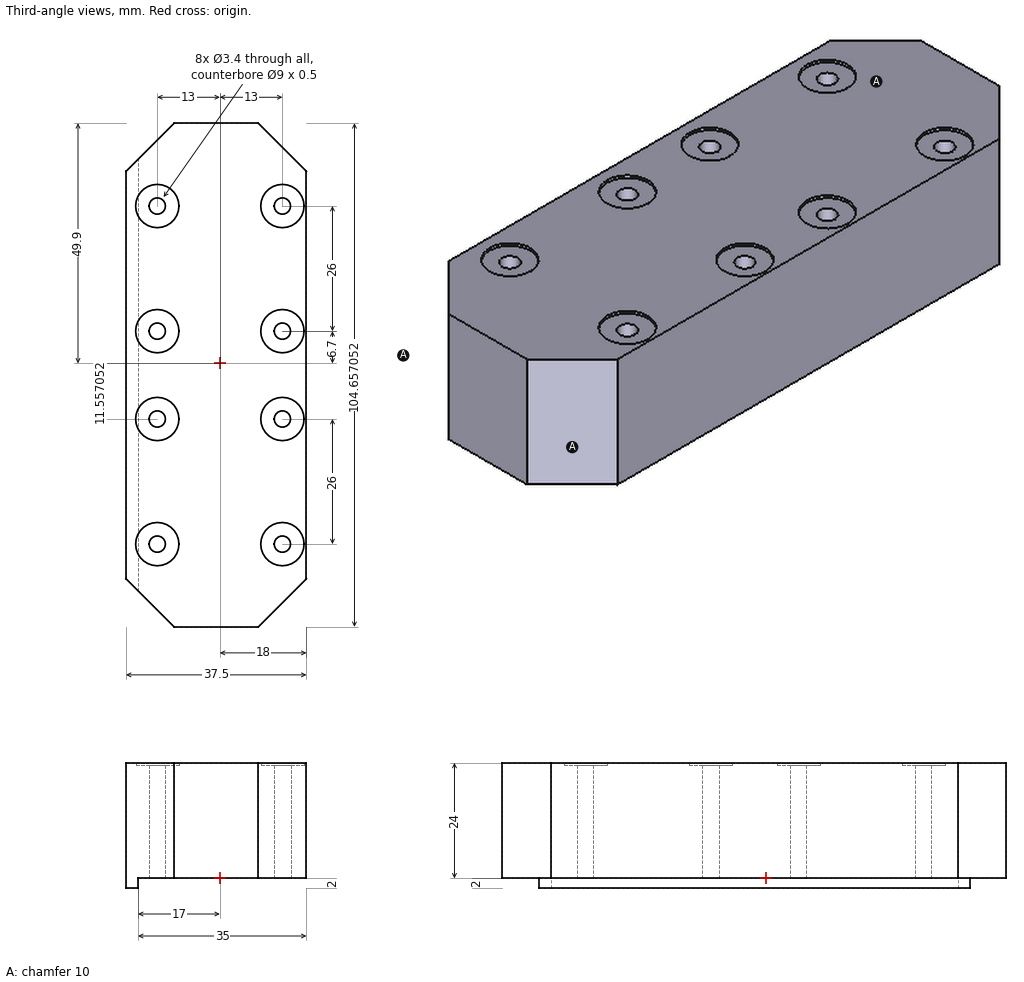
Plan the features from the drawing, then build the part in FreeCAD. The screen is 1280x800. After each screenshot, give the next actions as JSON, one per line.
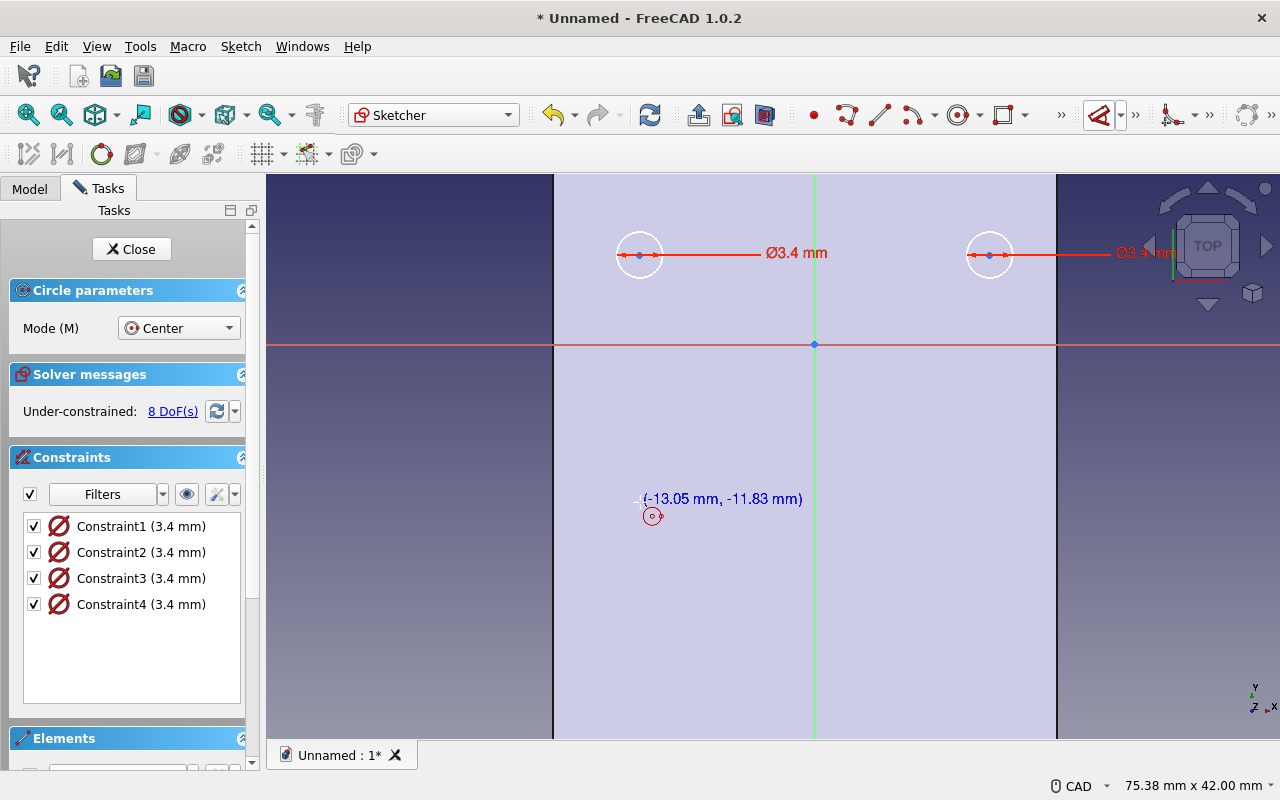
{"action": "left_click", "coordinate": [640, 500]}
{"action": "mouse_move", "coordinate": [656, 484]}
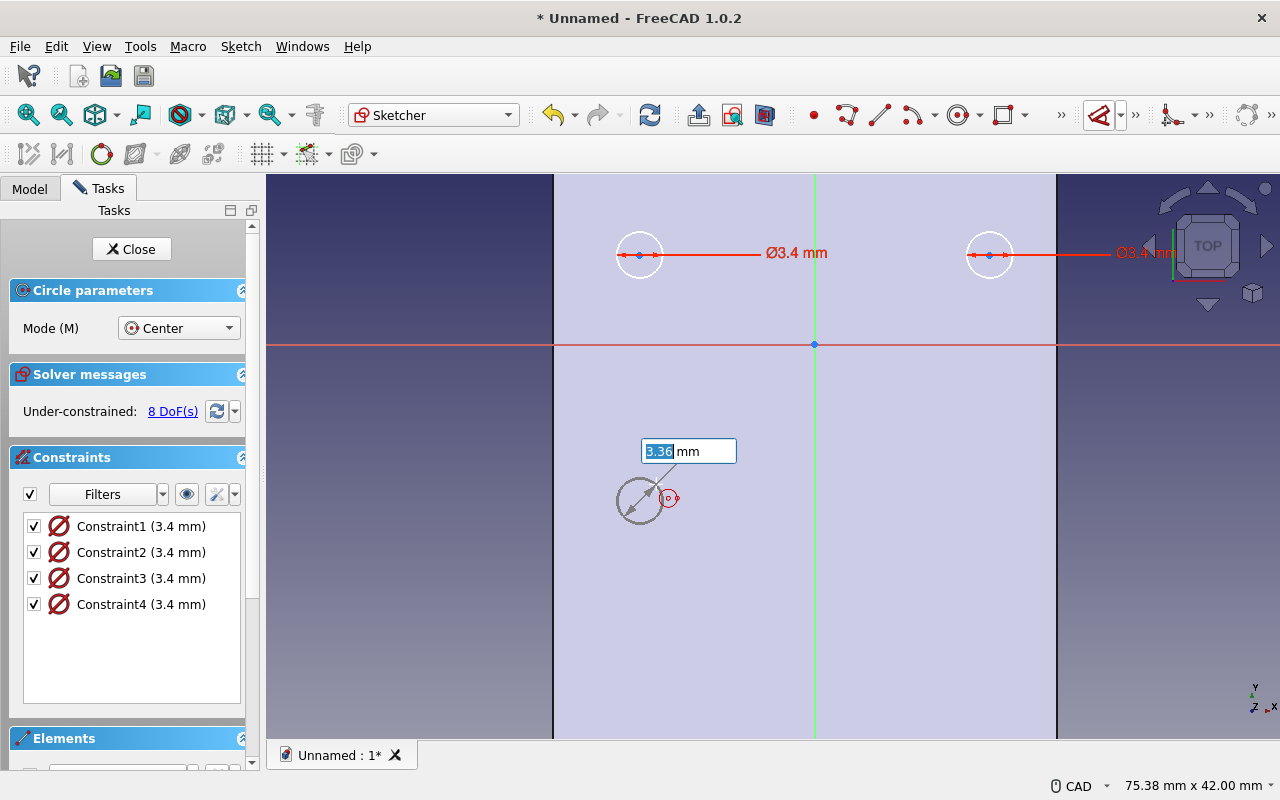
{"action": "type", "text": "3.4"}
{"action": "key", "text": "Return"}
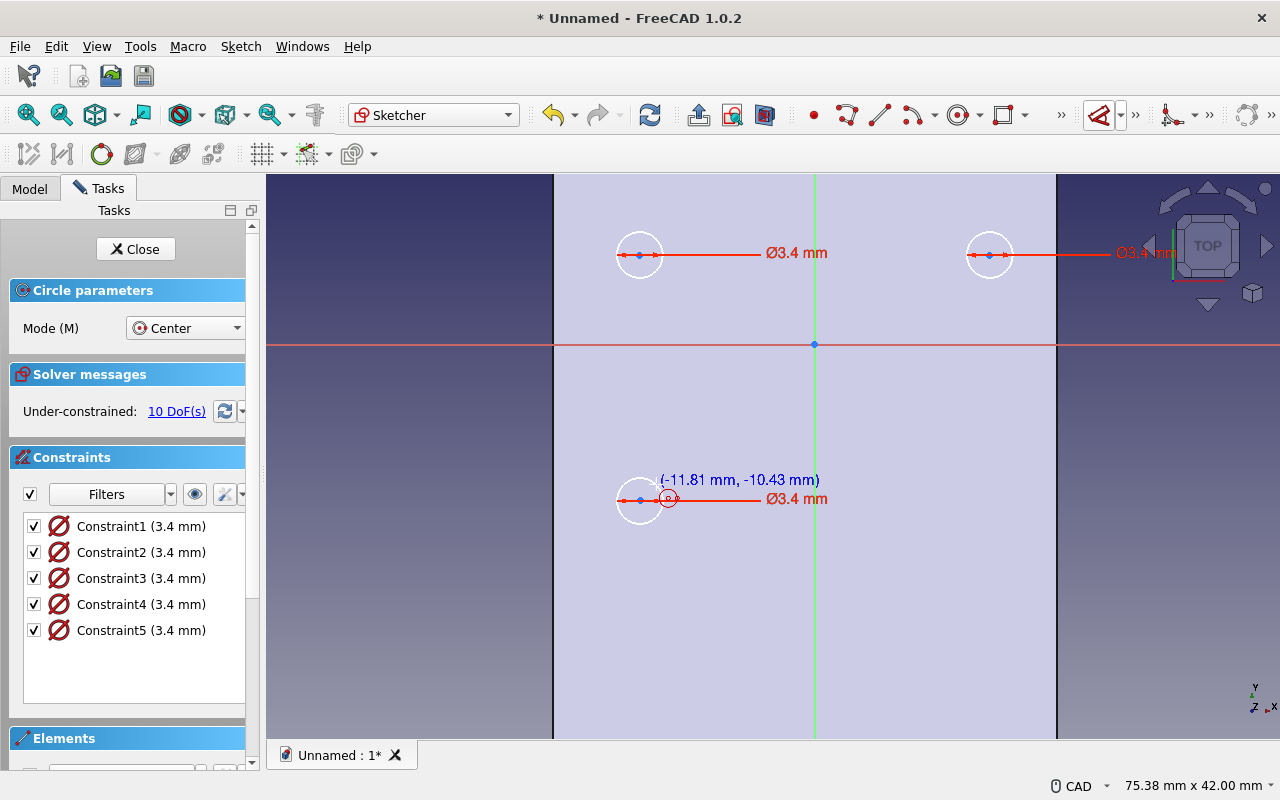
{"action": "left_click", "coordinate": [990, 500]}
{"action": "mouse_move", "coordinate": [1006, 484]}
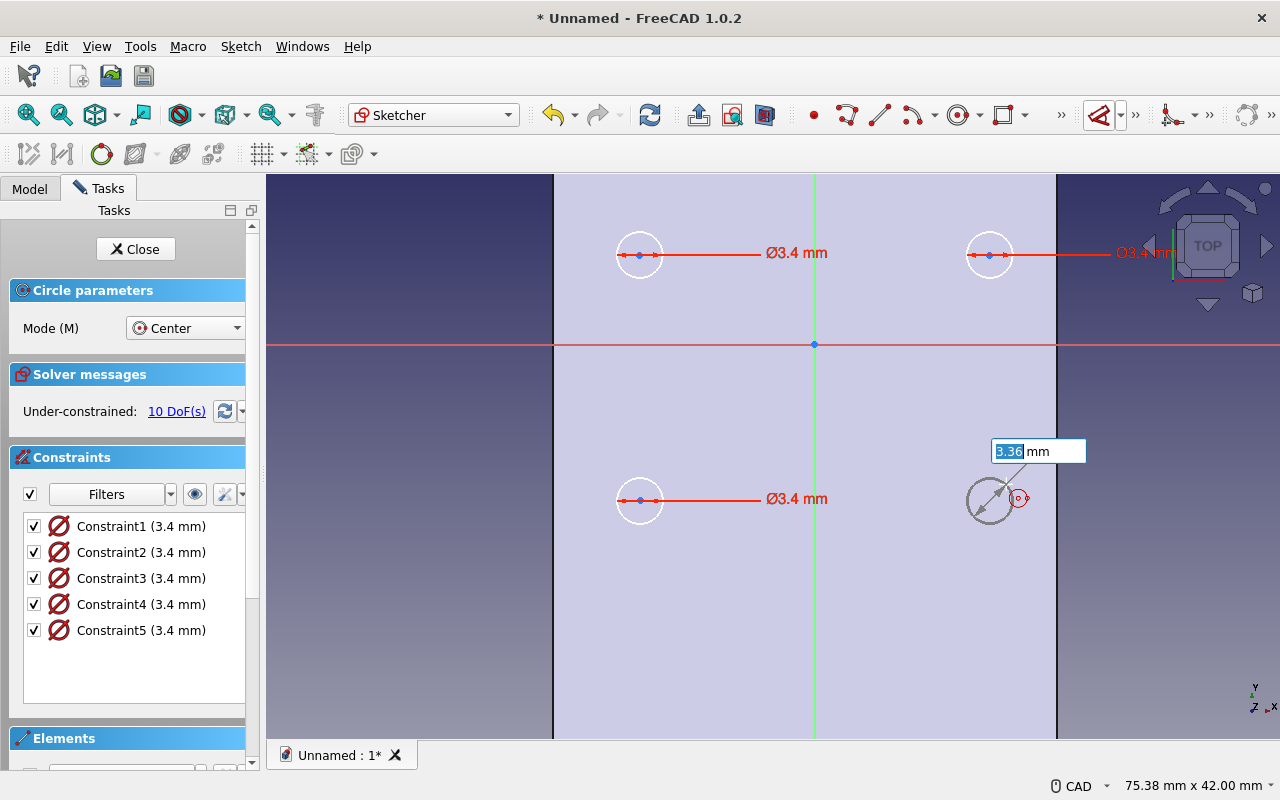
{"action": "type", "text": "3.4"}
{"action": "key", "text": "Return"}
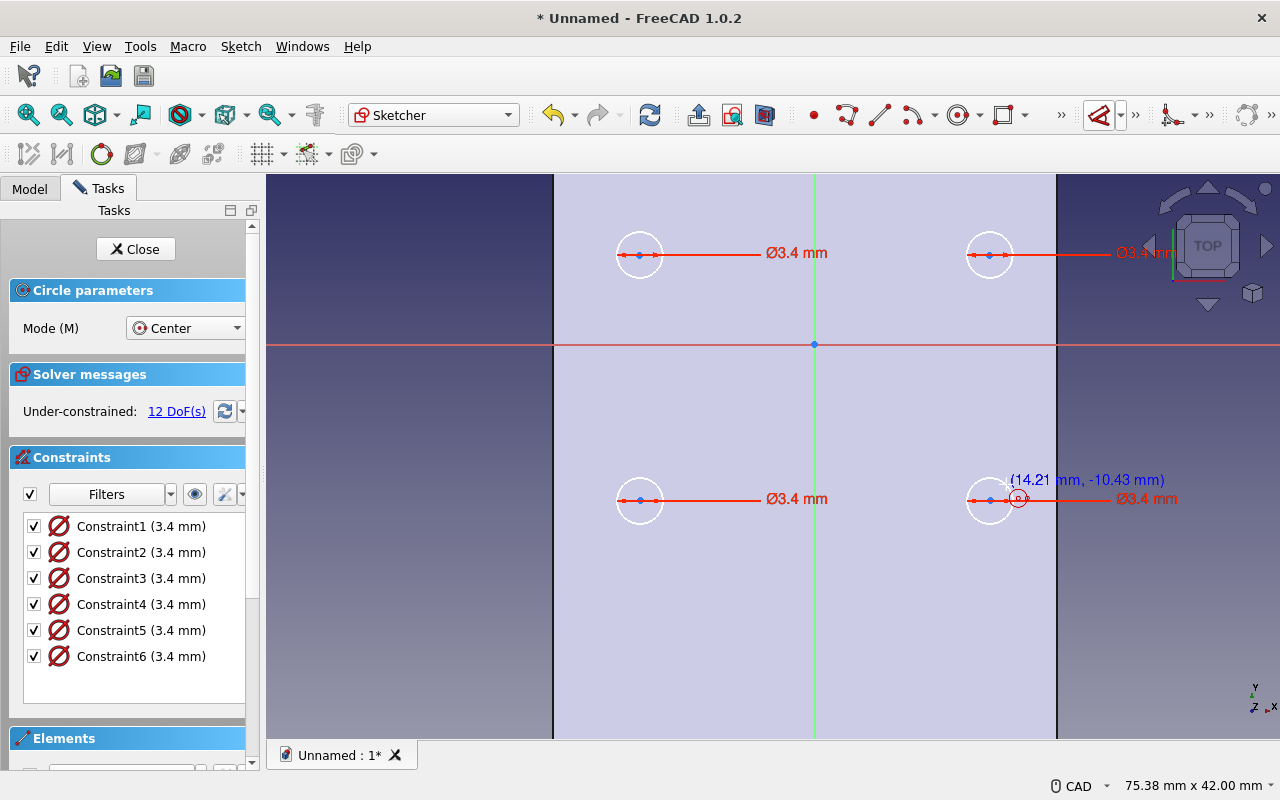
{"action": "scroll", "coordinate": [640, 503], "scroll_direction": "down", "scroll_amount": 5}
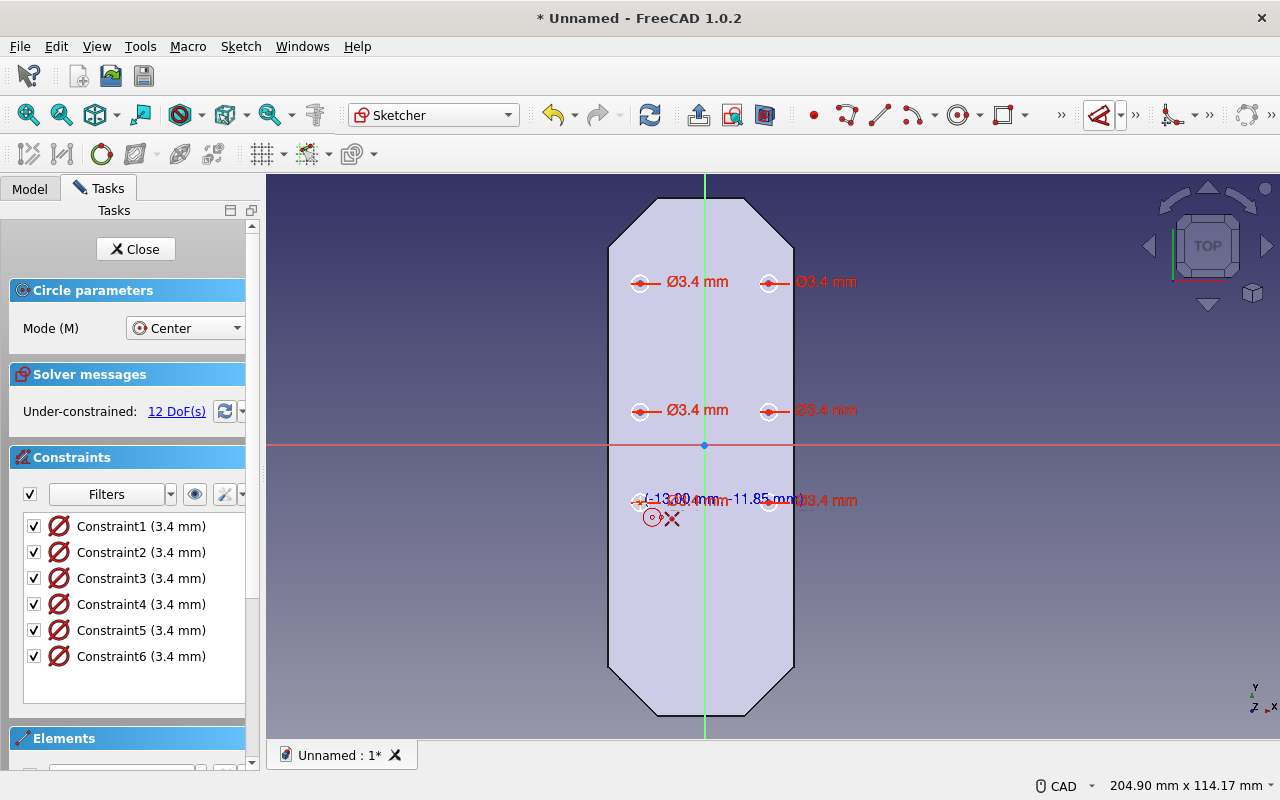
{"action": "scroll", "coordinate": [769, 631], "scroll_direction": "up", "scroll_amount": 5}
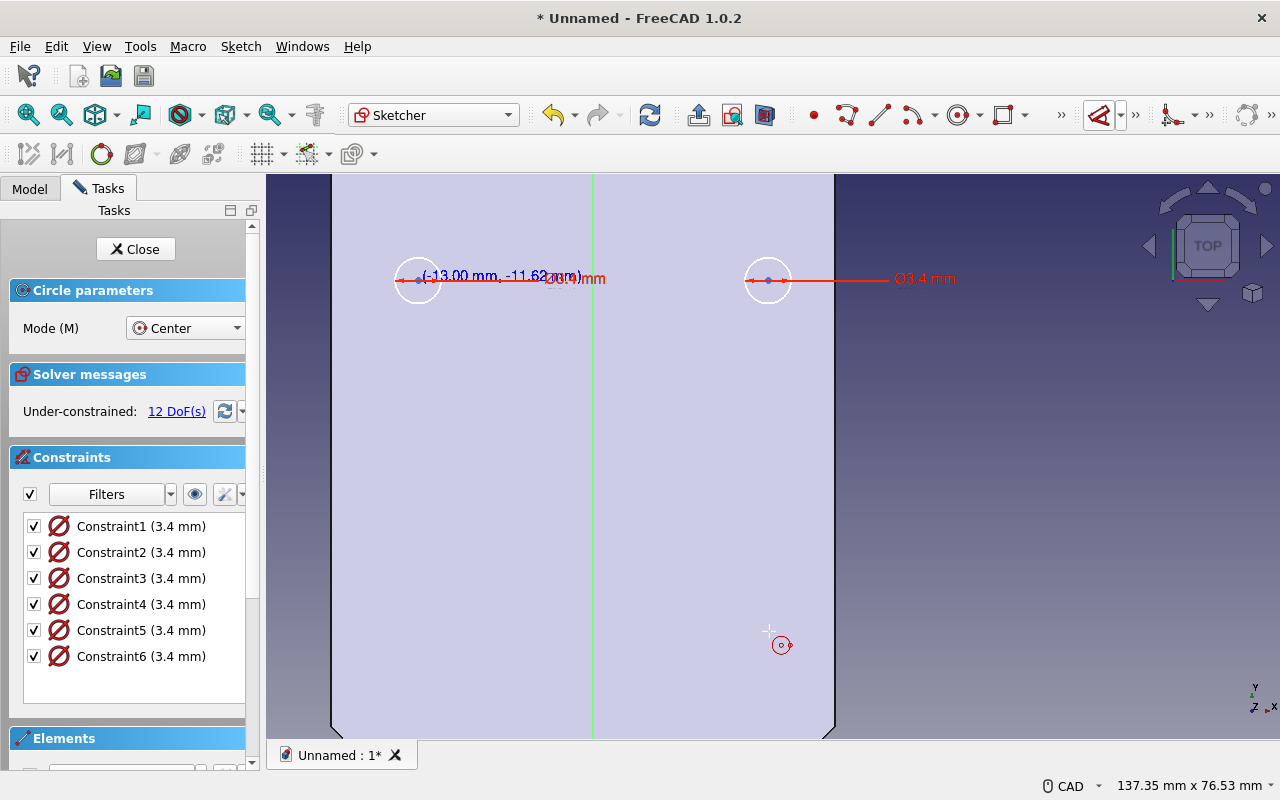
{"action": "left_click", "coordinate": [768, 630]}
{"action": "mouse_move", "coordinate": [784, 613]}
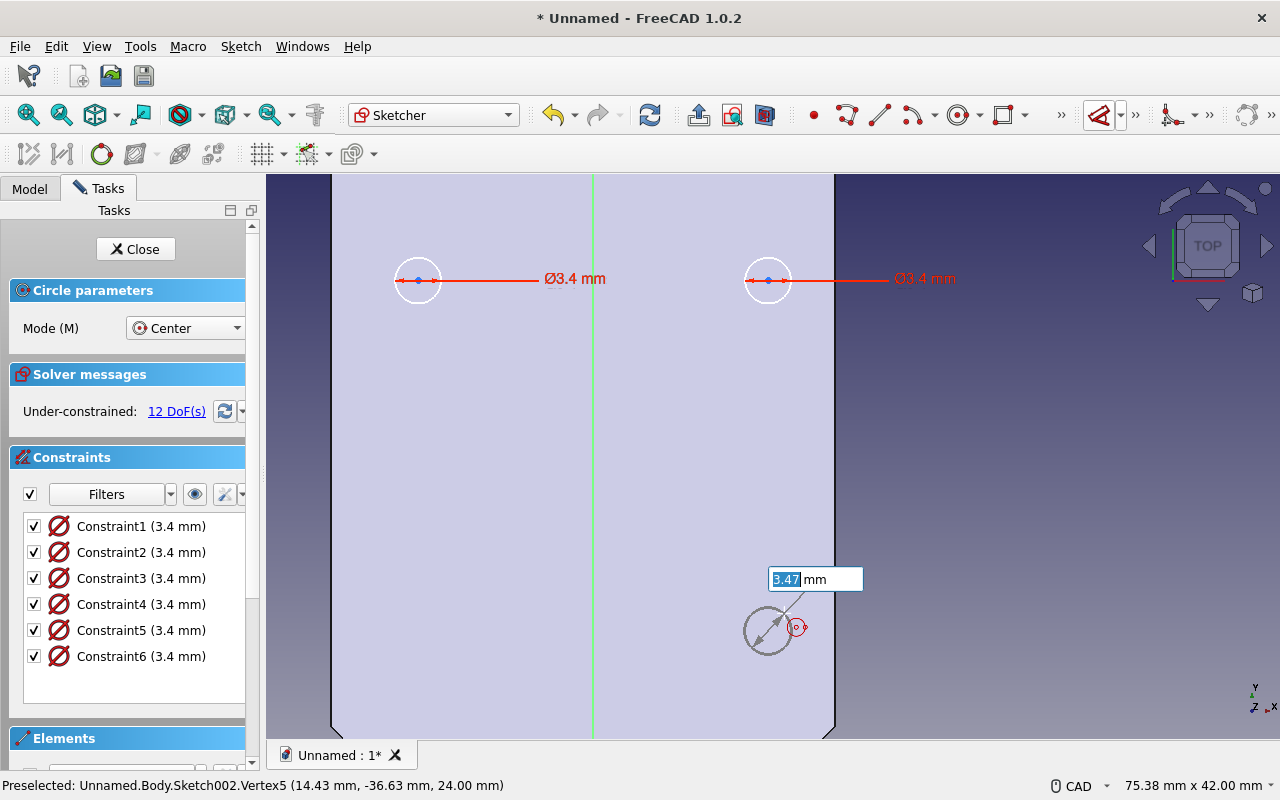
{"action": "type", "text": "3.4"}
{"action": "key", "text": "Return"}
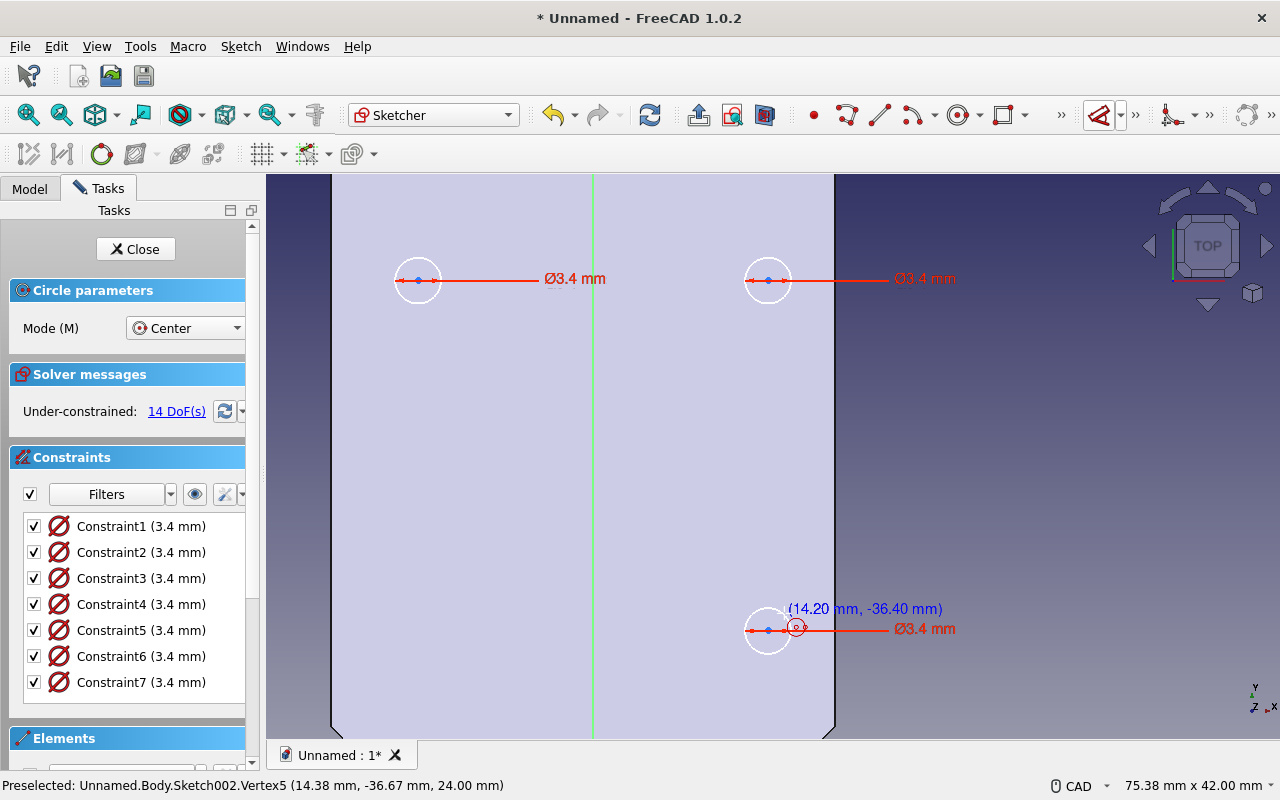
{"action": "left_click", "coordinate": [418, 630]}
{"action": "mouse_move", "coordinate": [434, 613]}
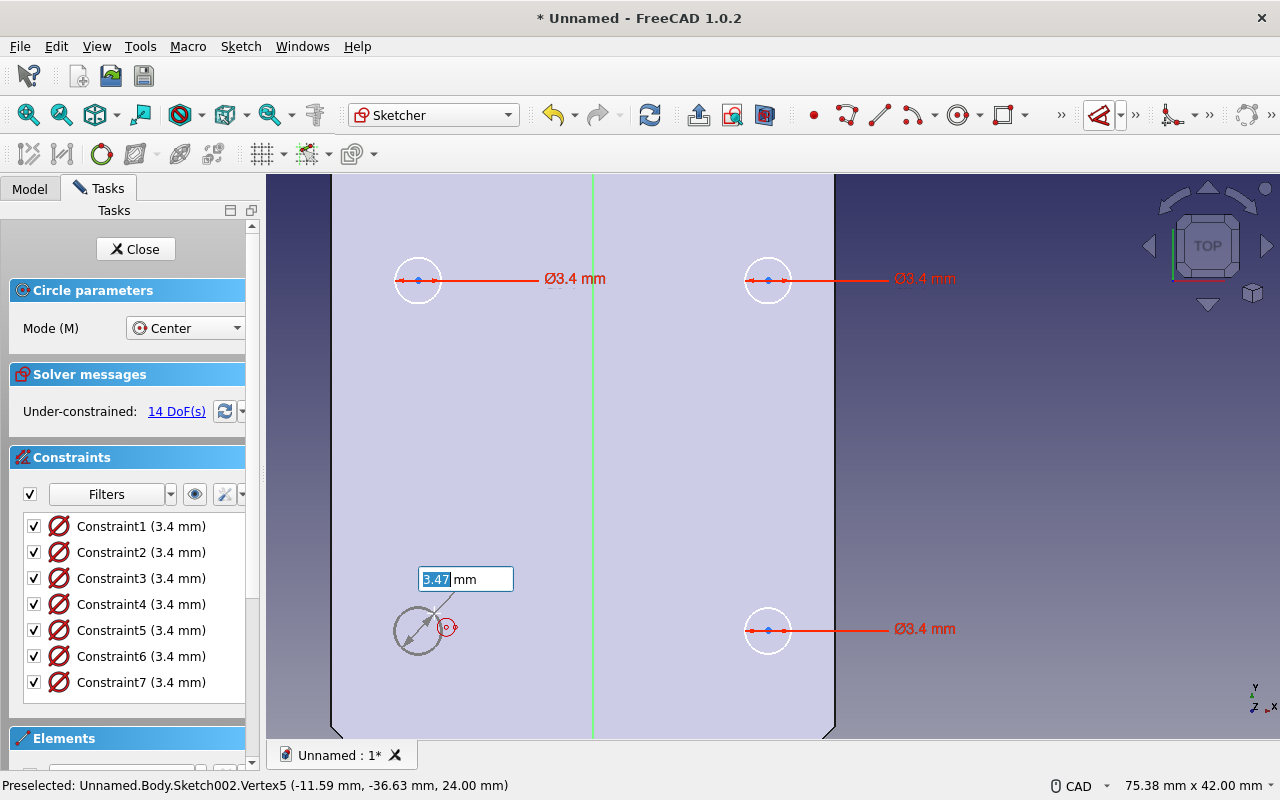
{"action": "type", "text": "3.4"}
{"action": "key", "text": "Return"}
{"action": "key", "text": "Escape"}